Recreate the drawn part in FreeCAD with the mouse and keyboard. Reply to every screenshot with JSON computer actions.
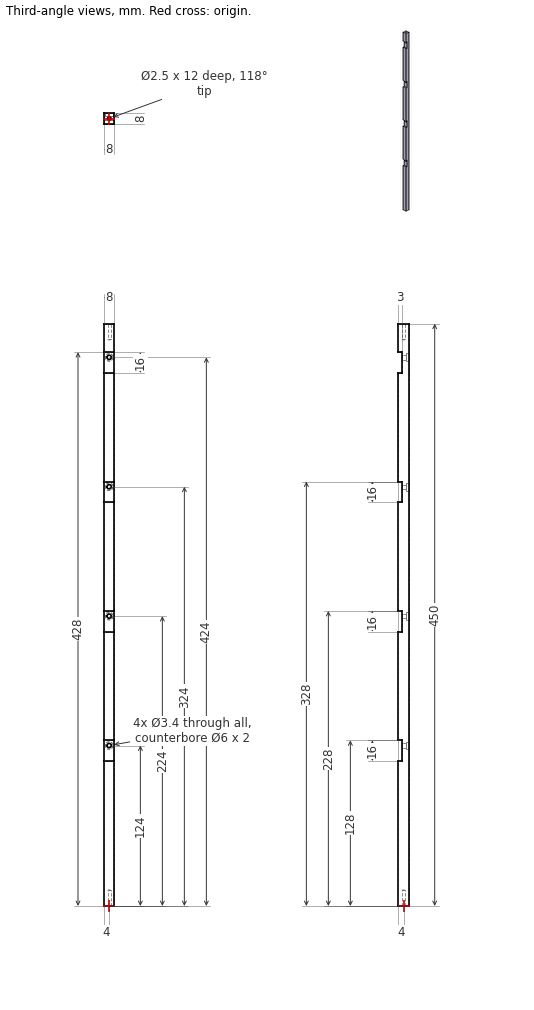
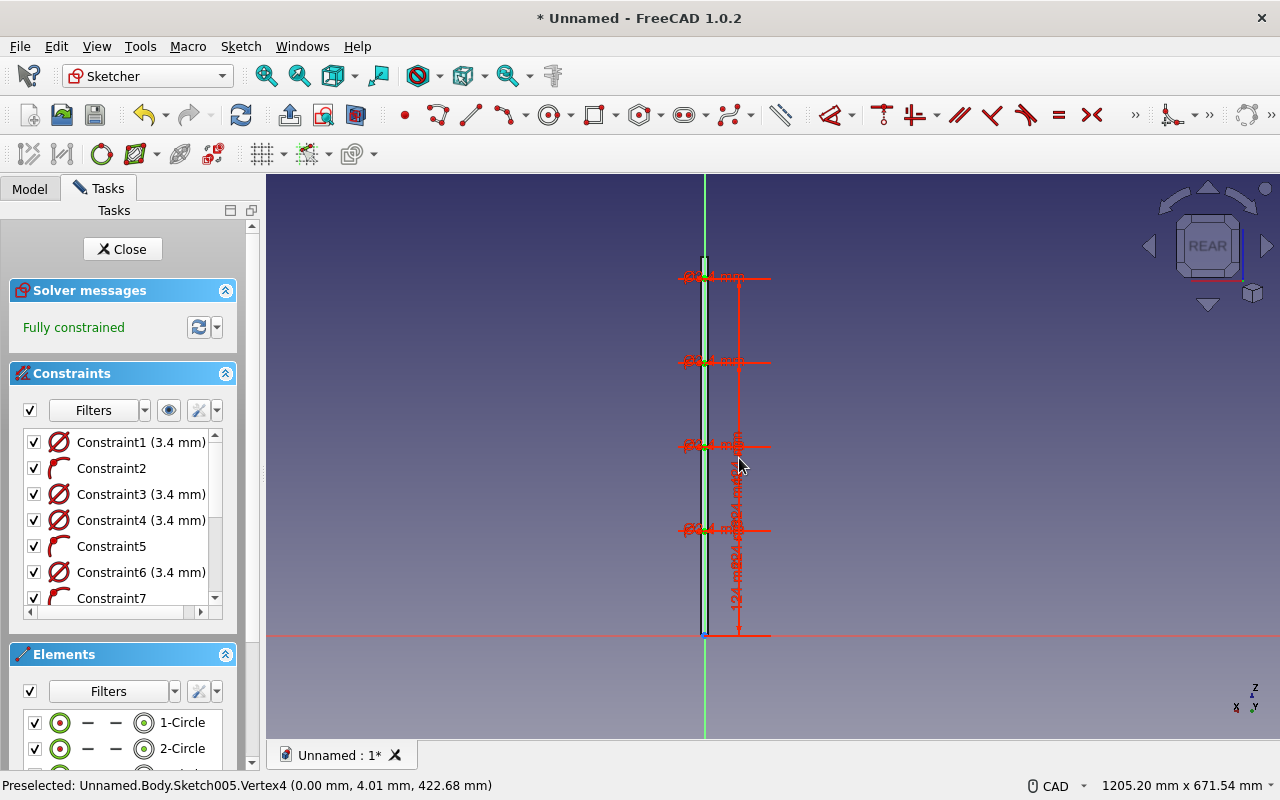
{"action": "left_click", "coordinate": [123, 249]}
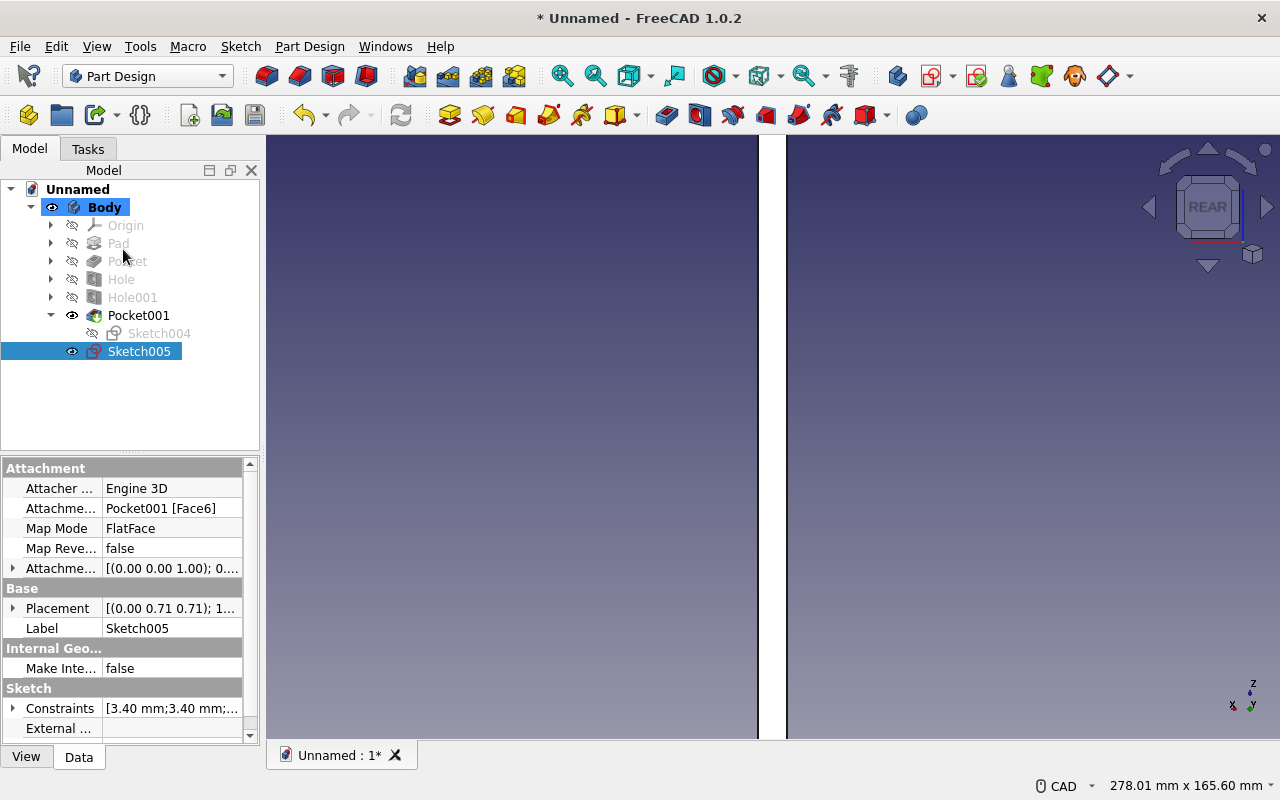
{"action": "left_click", "coordinate": [700, 116]}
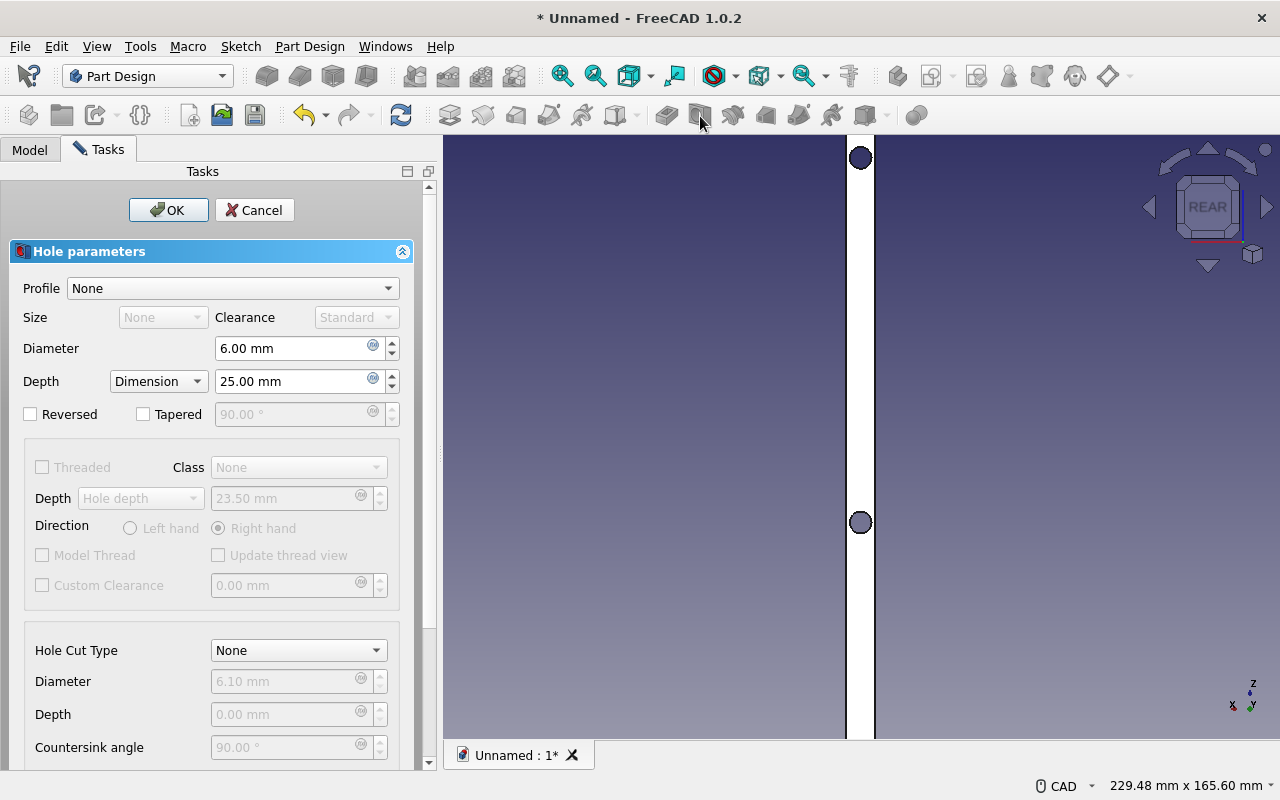
{"action": "triple_click", "coordinate": [300, 348]}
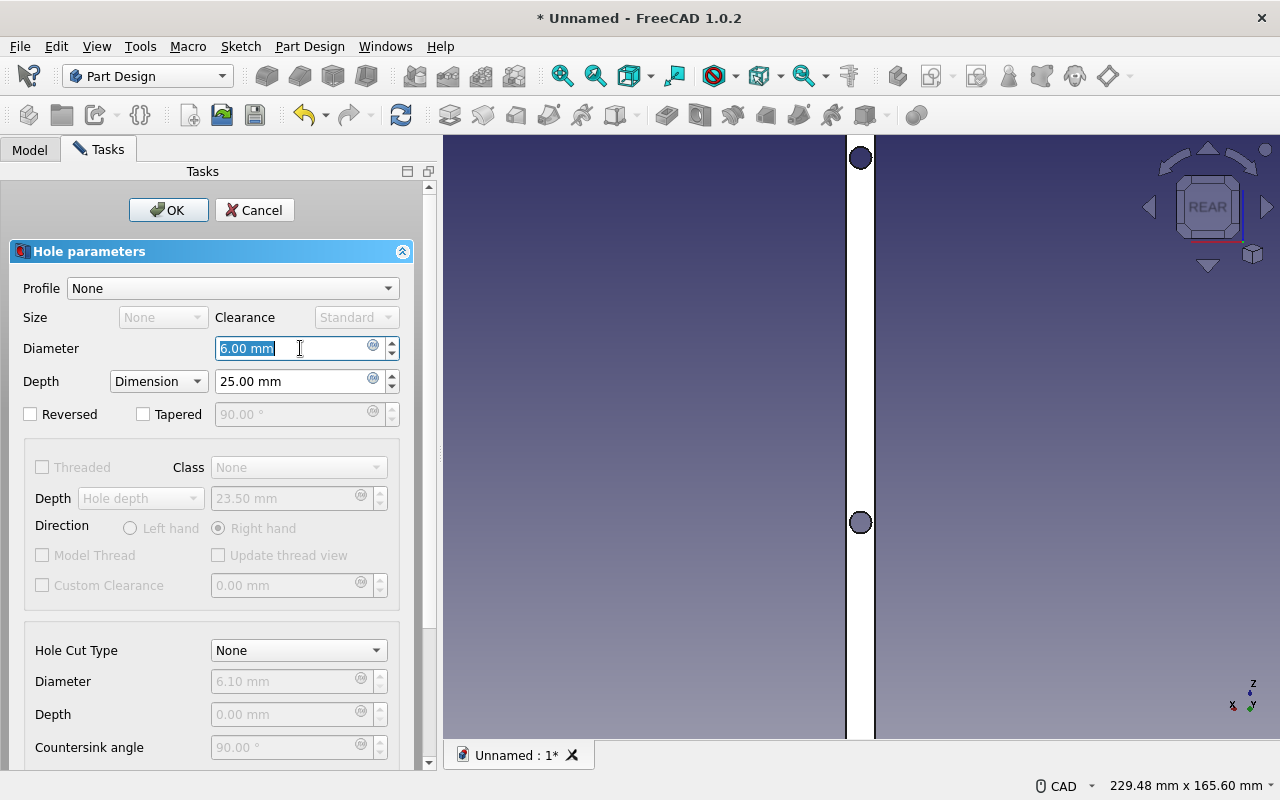
{"action": "type", "text": "3.4"}
{"action": "key", "text": "Tab"}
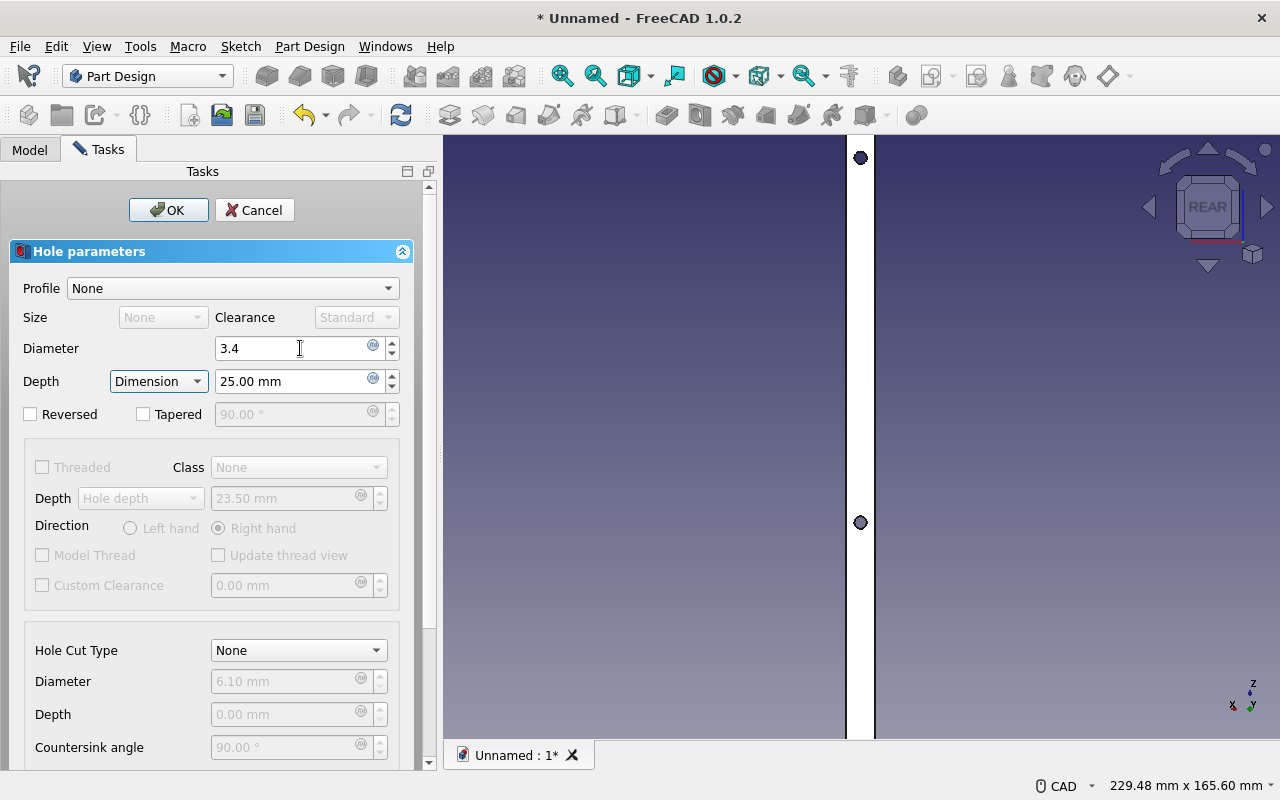
{"action": "left_click", "coordinate": [160, 382]}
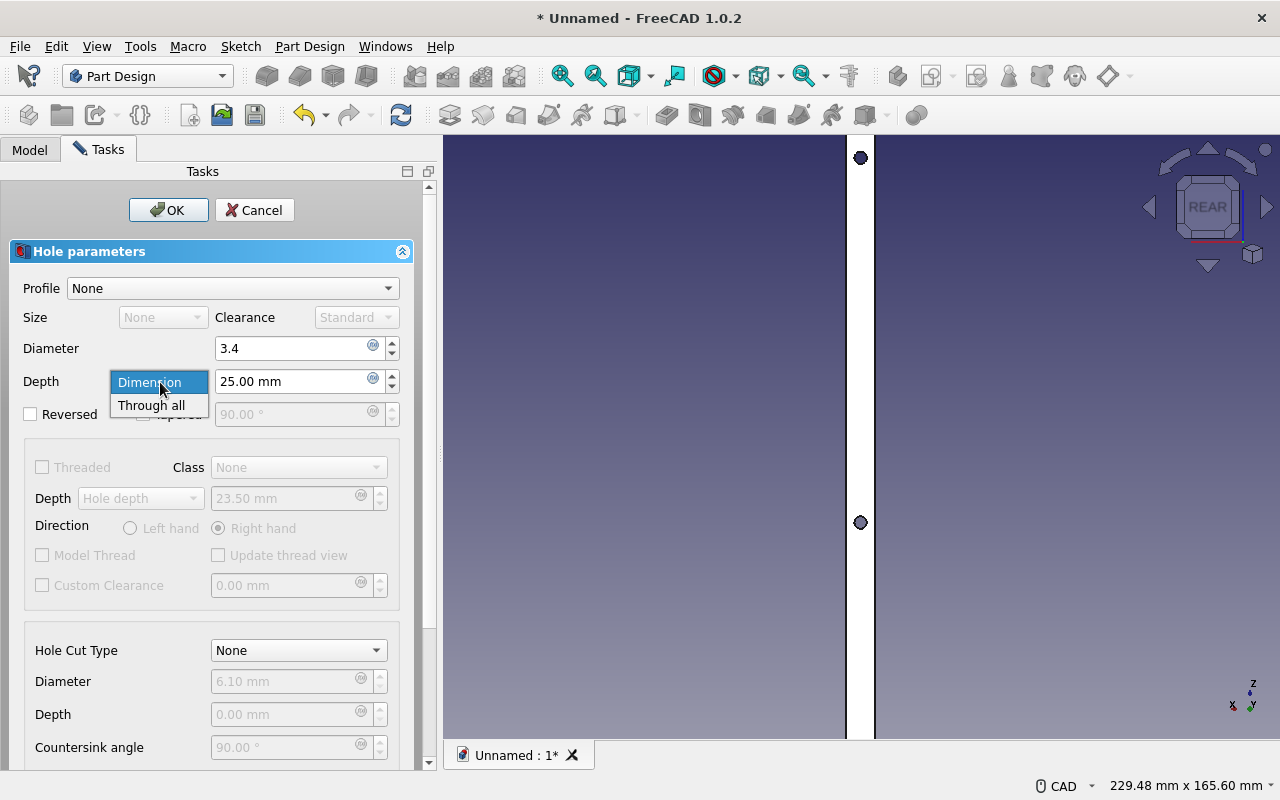
{"action": "left_click", "coordinate": [158, 406]}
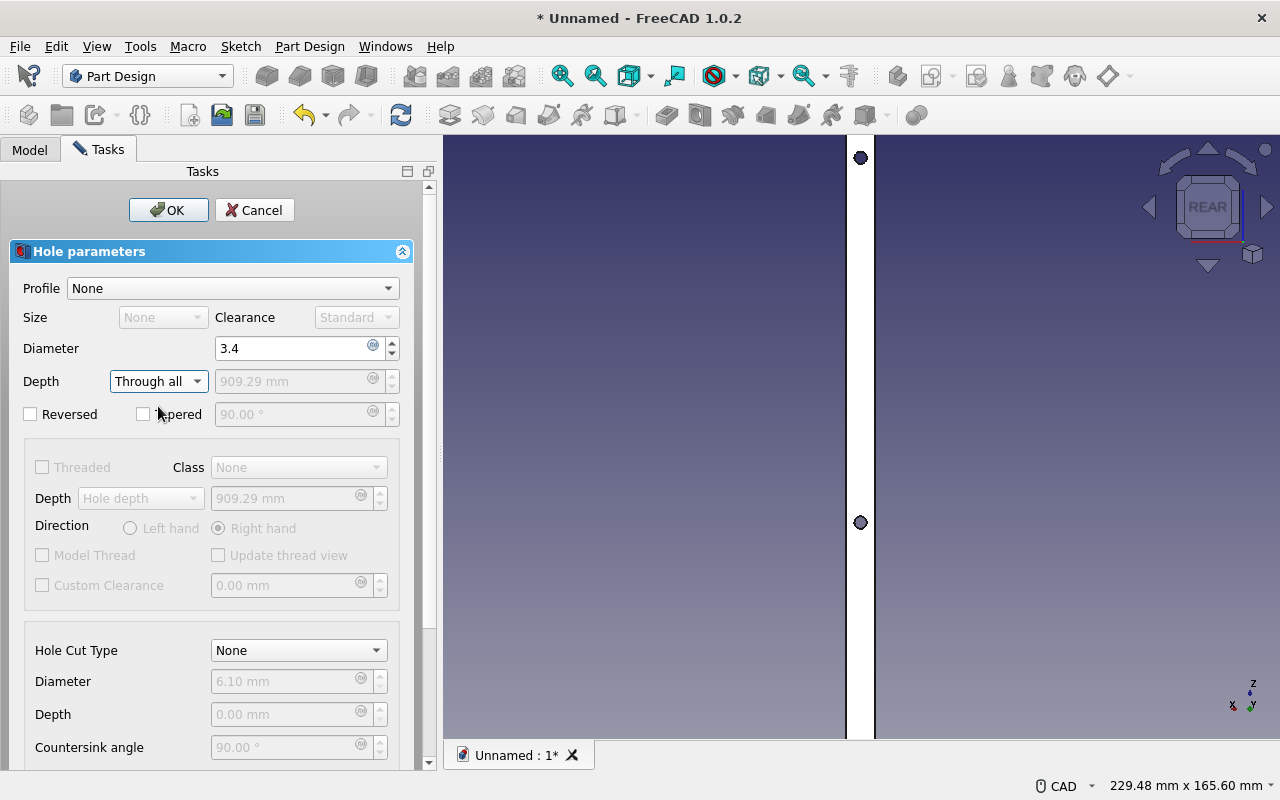
{"action": "left_click", "coordinate": [300, 650]}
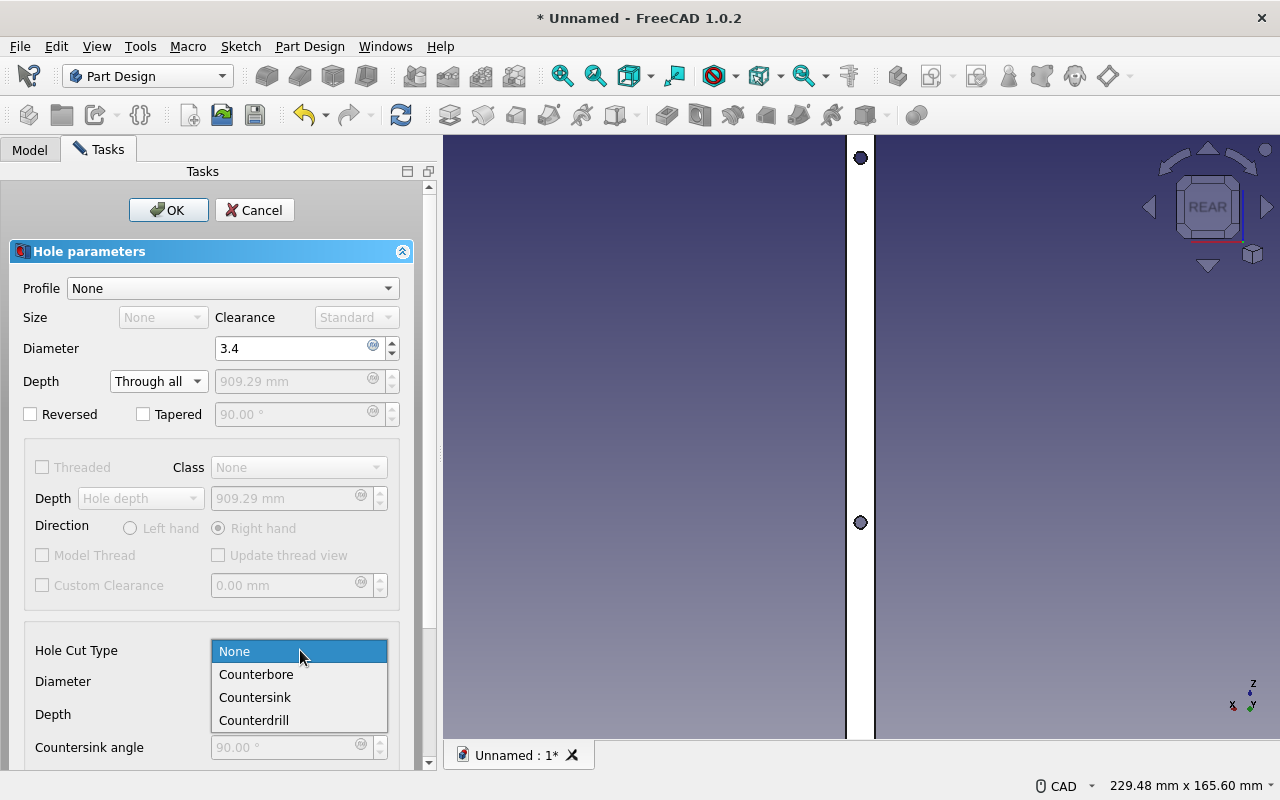
{"action": "left_click", "coordinate": [298, 674]}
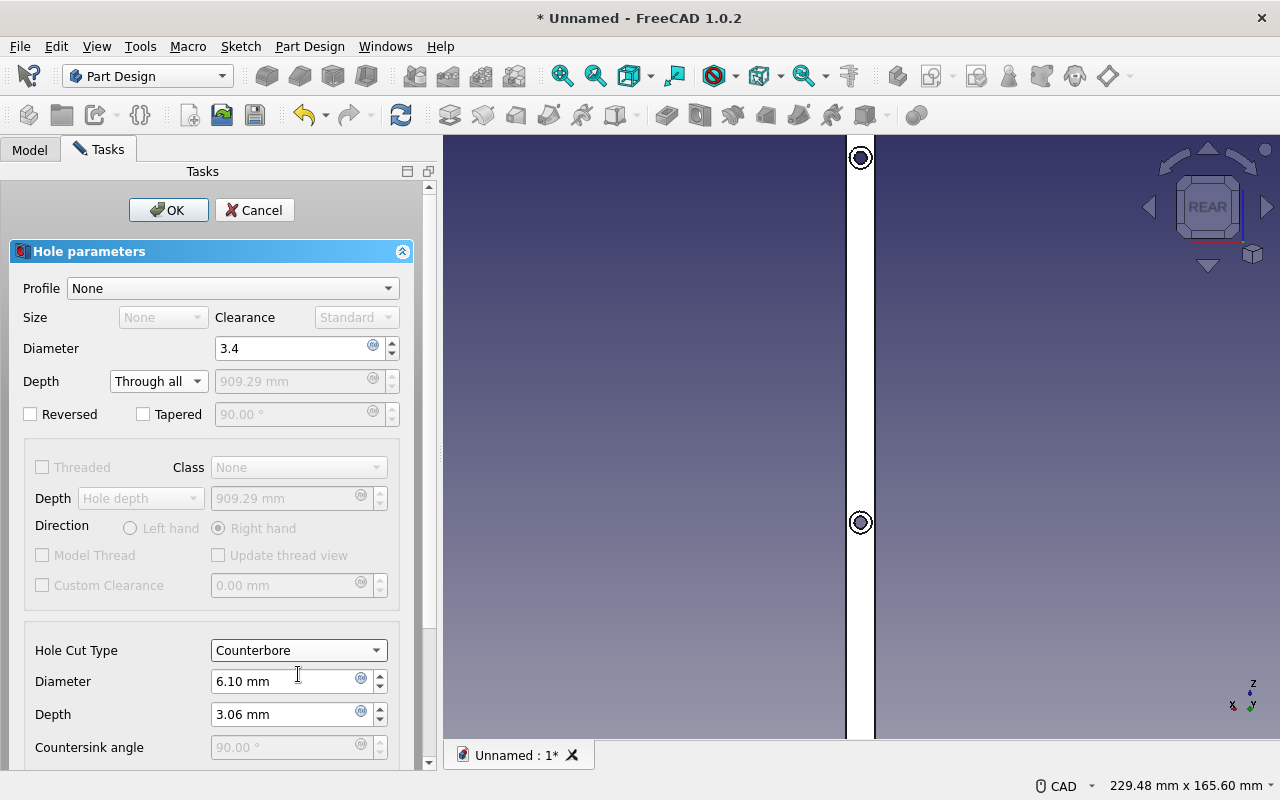
{"action": "triple_click", "coordinate": [292, 682]}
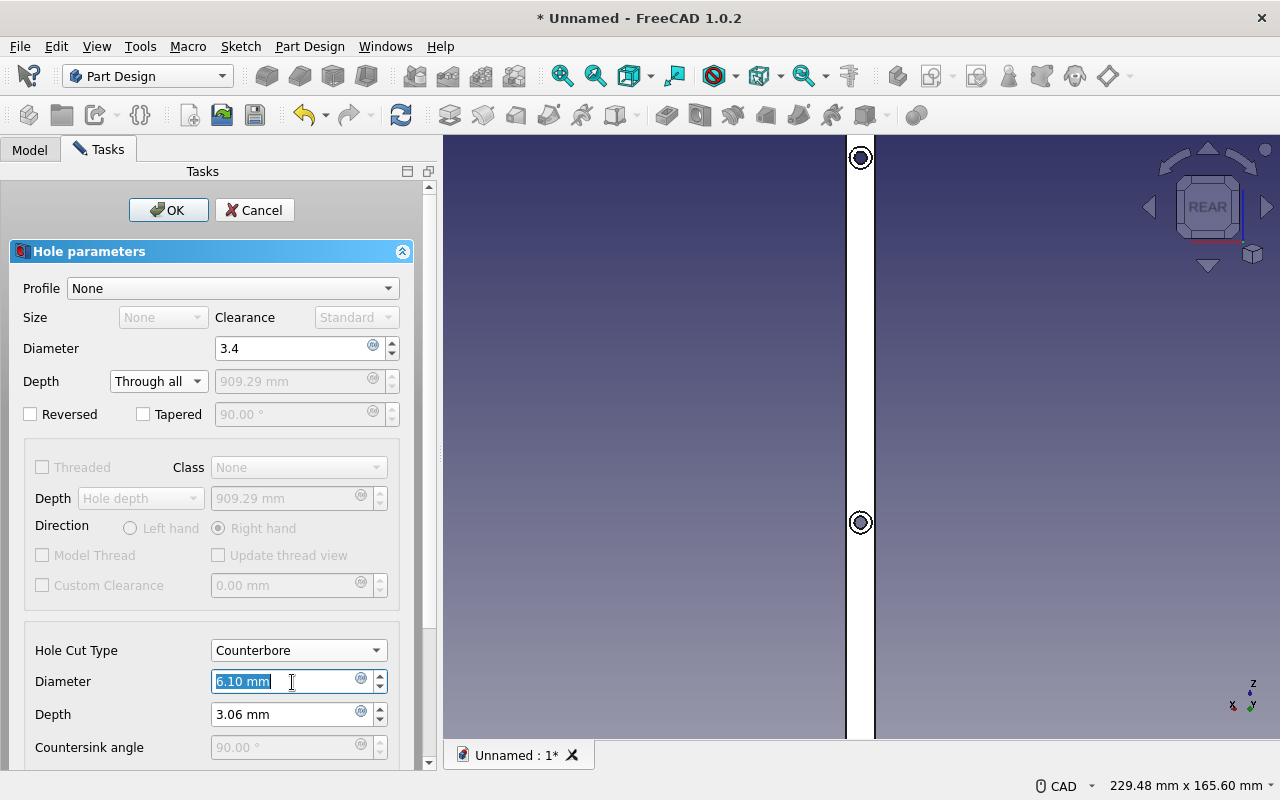
{"action": "type", "text": "6"}
{"action": "key", "text": "Tab"}